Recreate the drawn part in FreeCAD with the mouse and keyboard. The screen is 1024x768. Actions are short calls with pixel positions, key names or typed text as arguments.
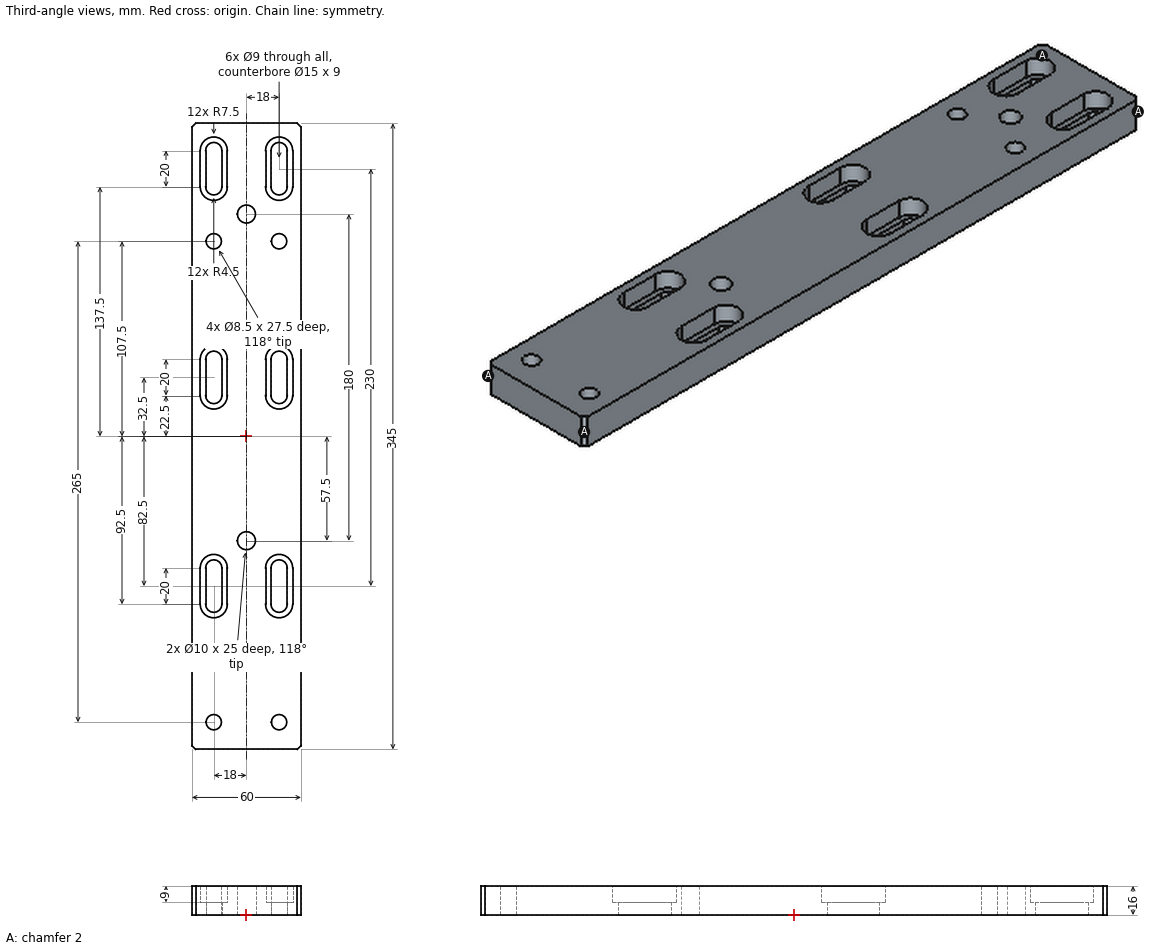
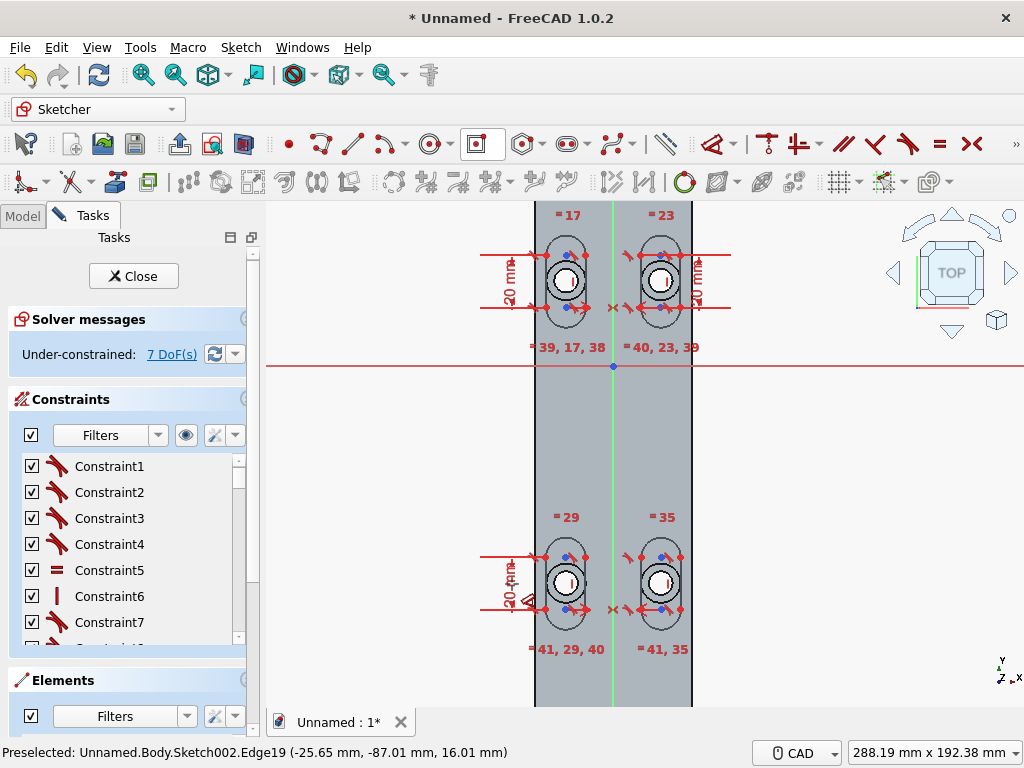
click(641, 594)
click(699, 584)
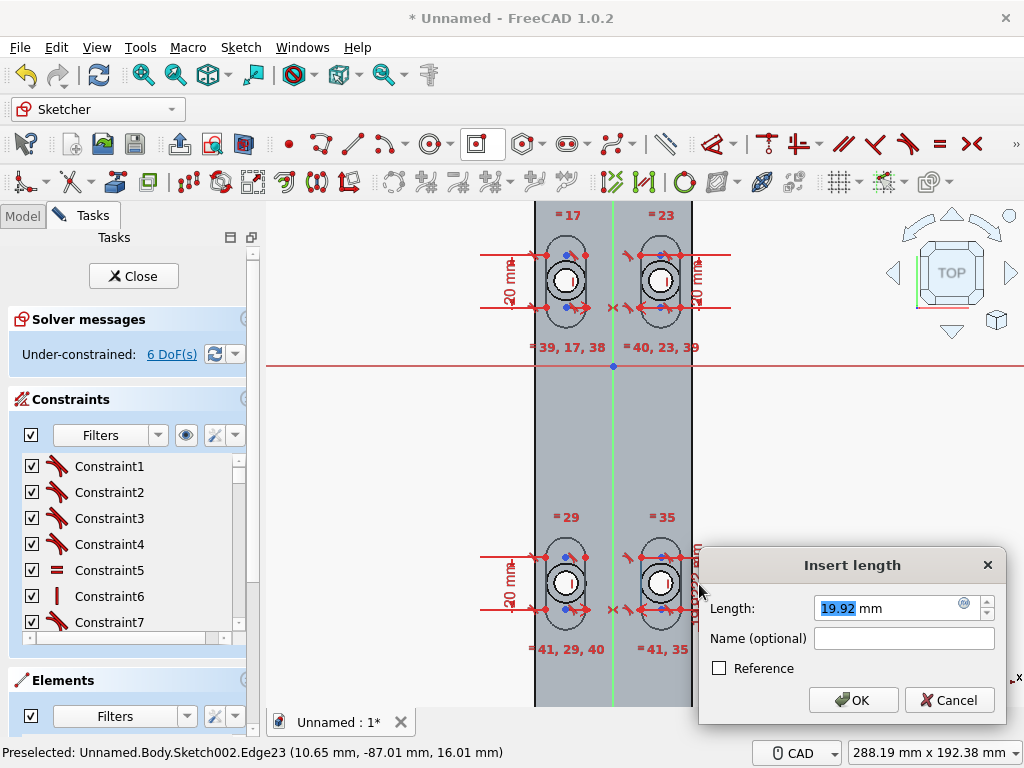
text(20)
key(Return)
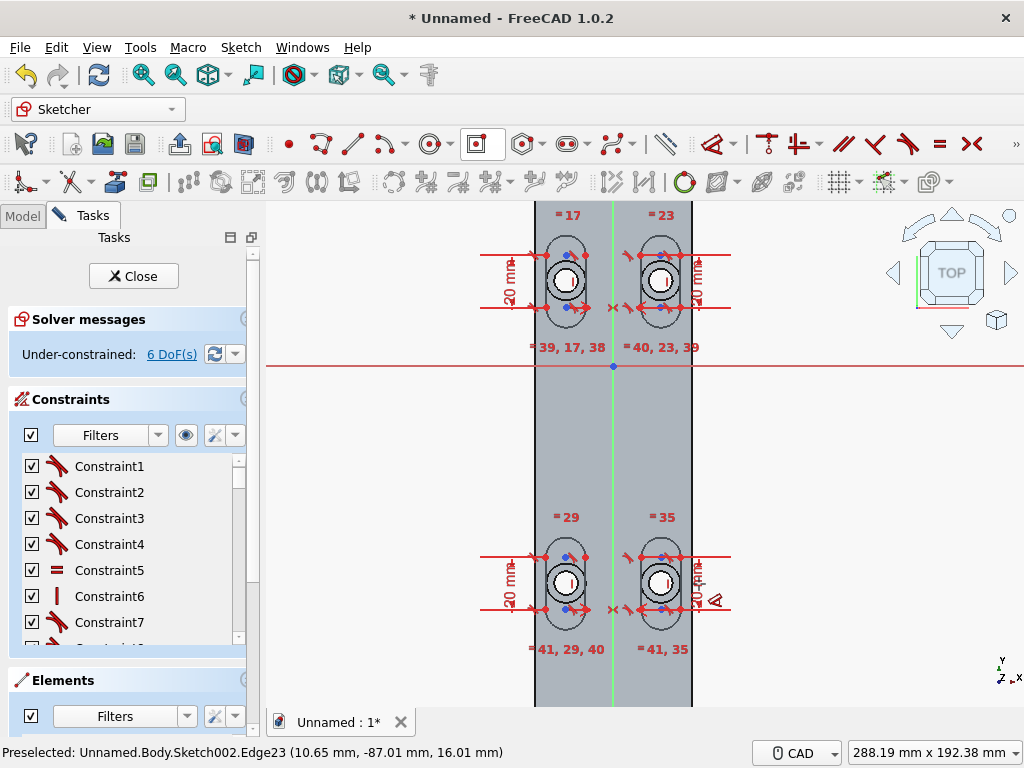
scroll(546, 595, down, 4)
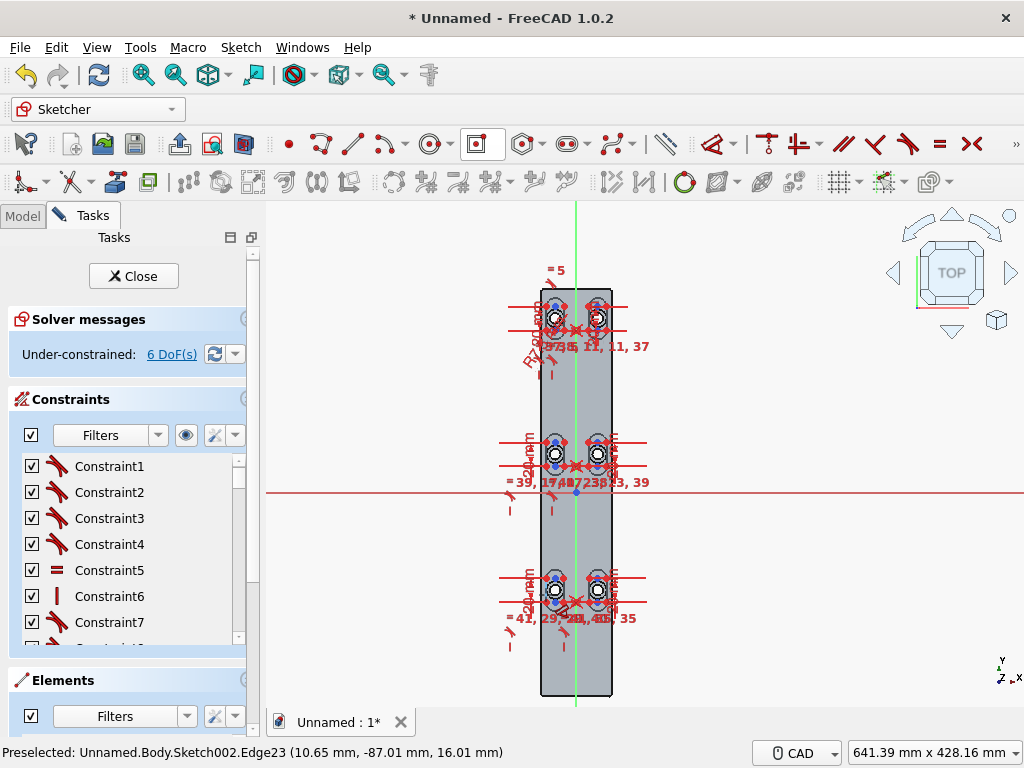
scroll(555, 331, up, 4)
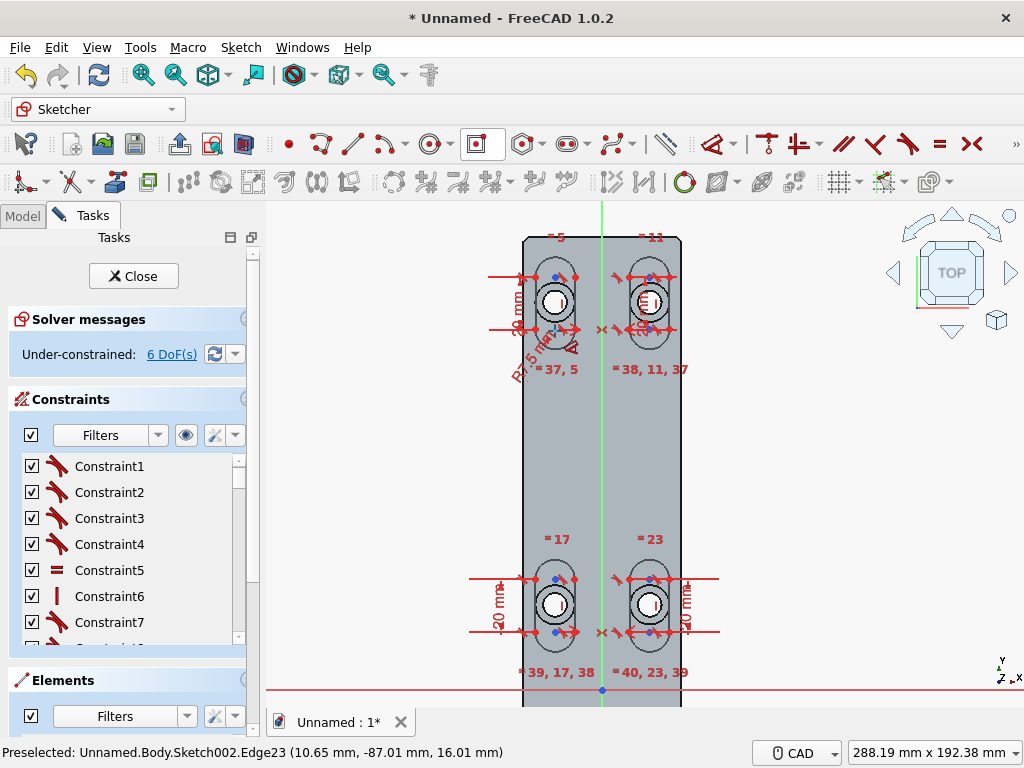
click(555, 330)
click(579, 248)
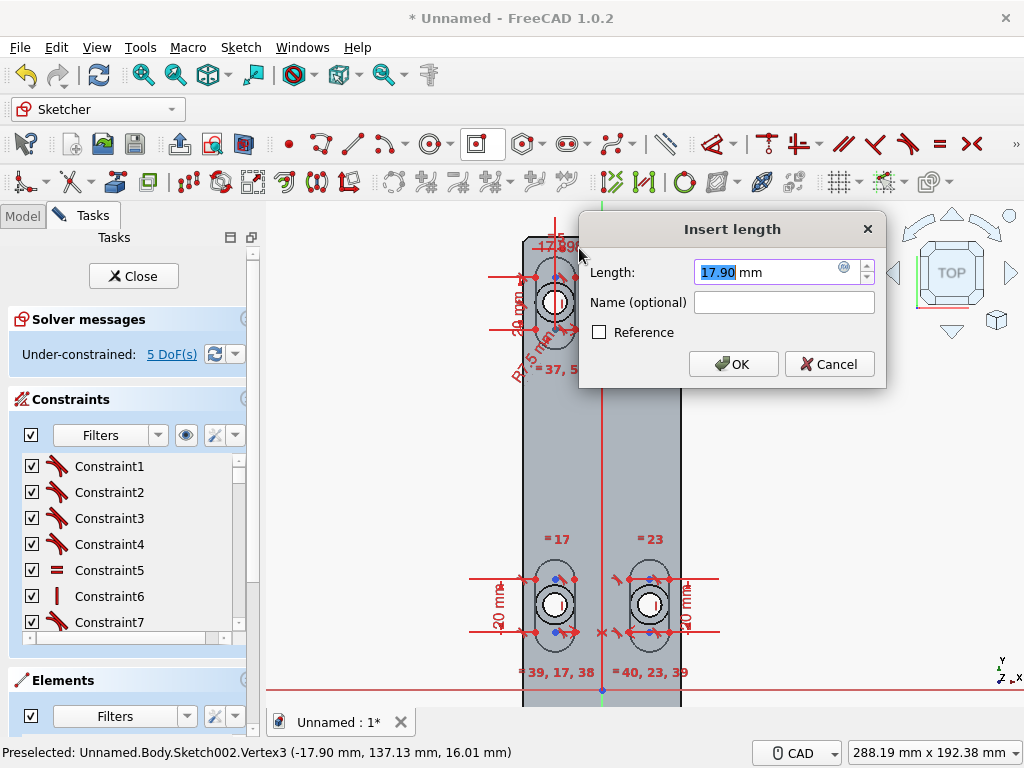
text(18)
key(Return)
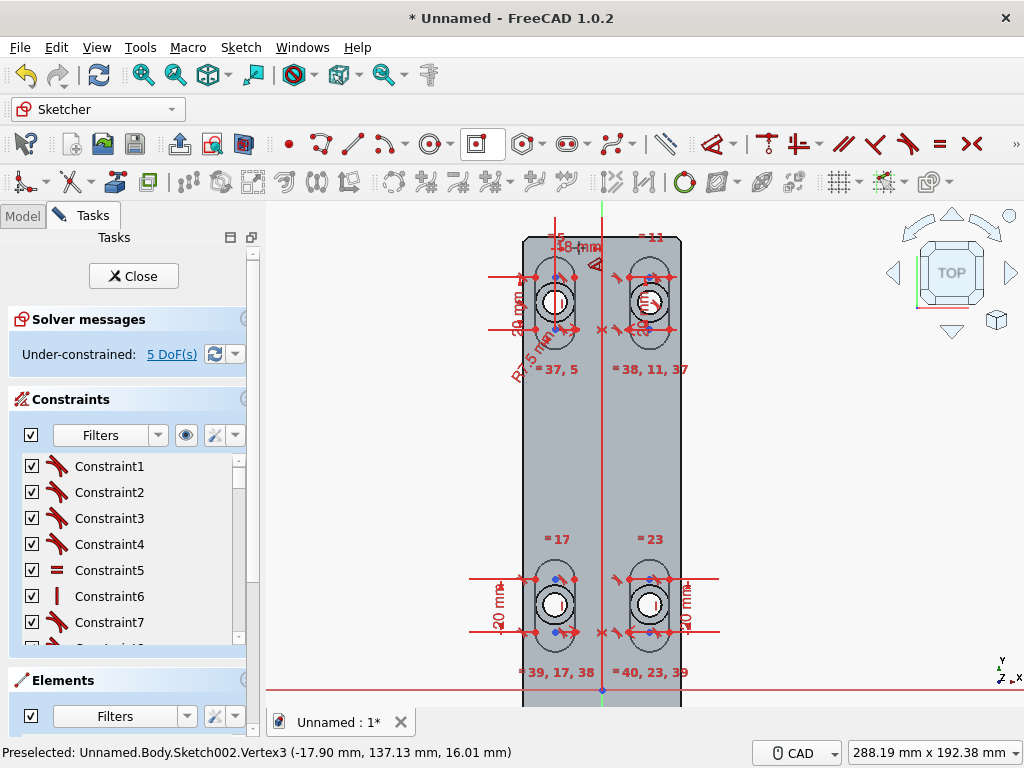
click(555, 632)
click(579, 550)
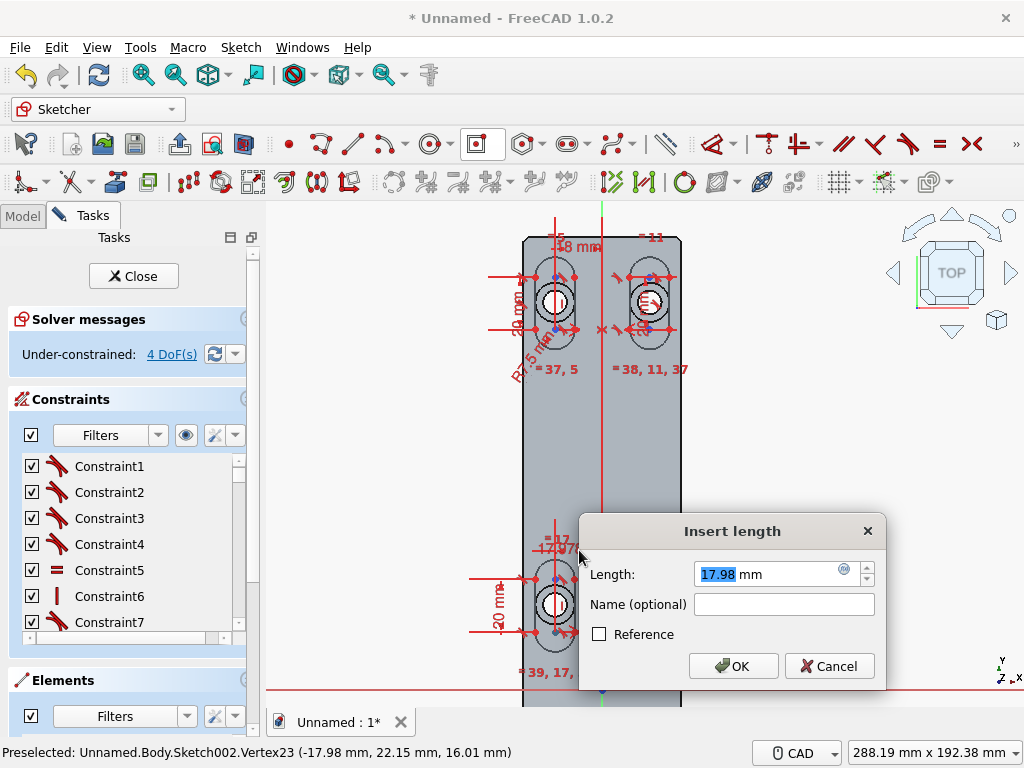
text(18)
key(Return)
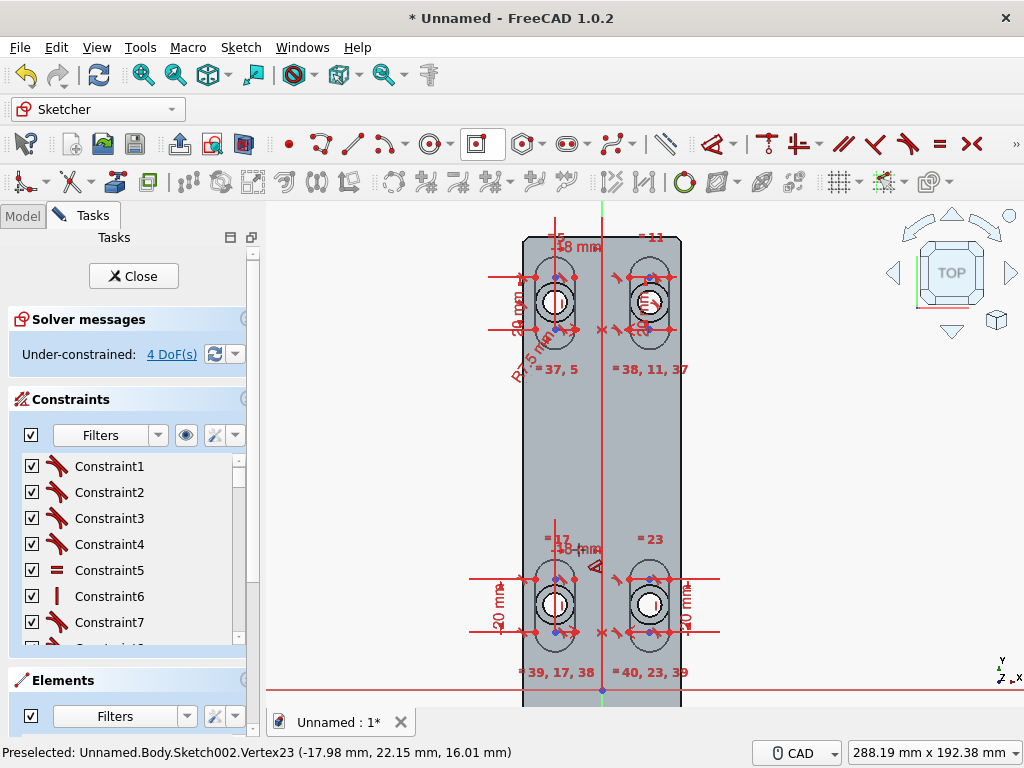
scroll(555, 331, down, 4)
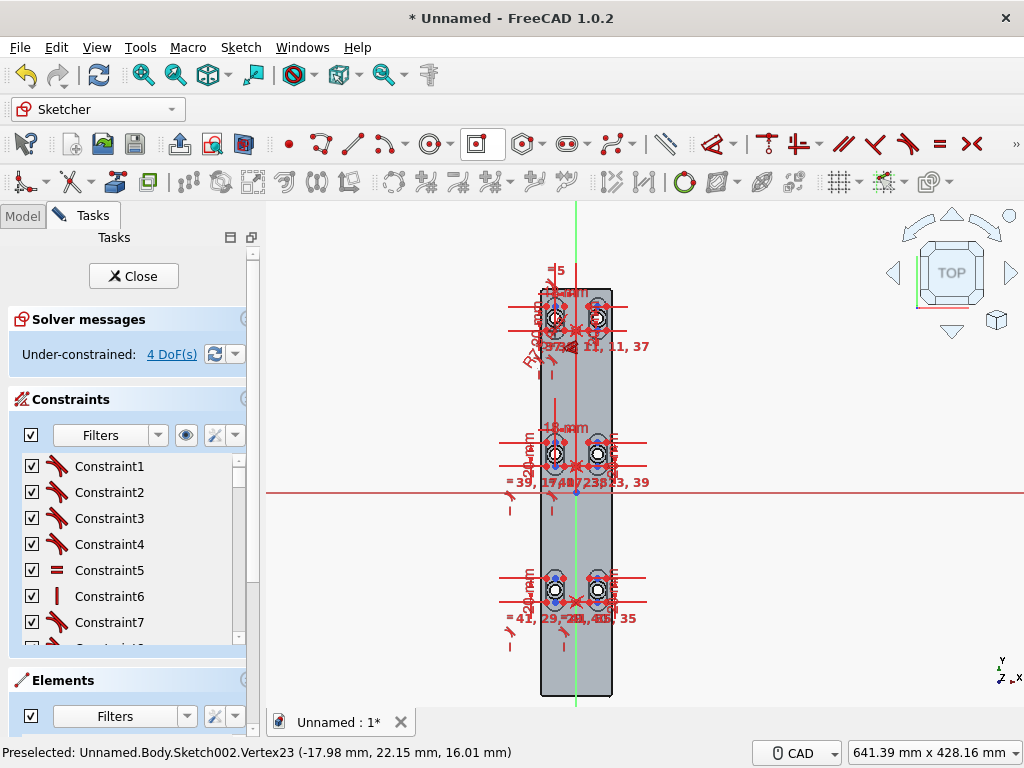
scroll(555, 602, up, 4)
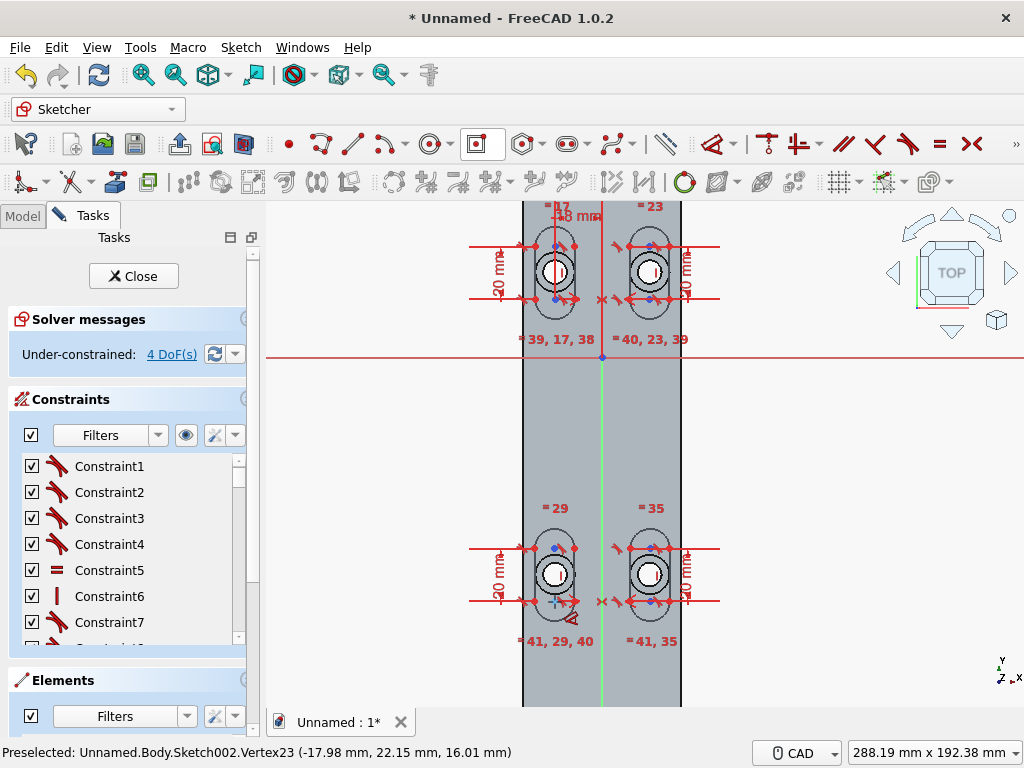
click(555, 601)
click(579, 635)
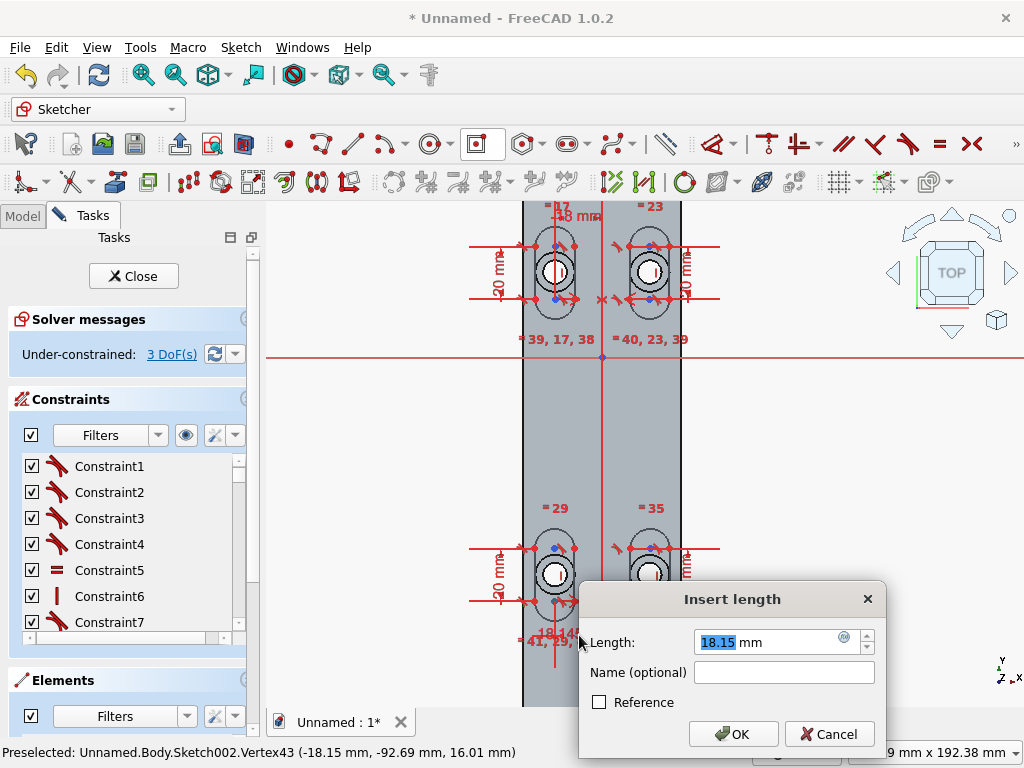
text(18)
key(Return)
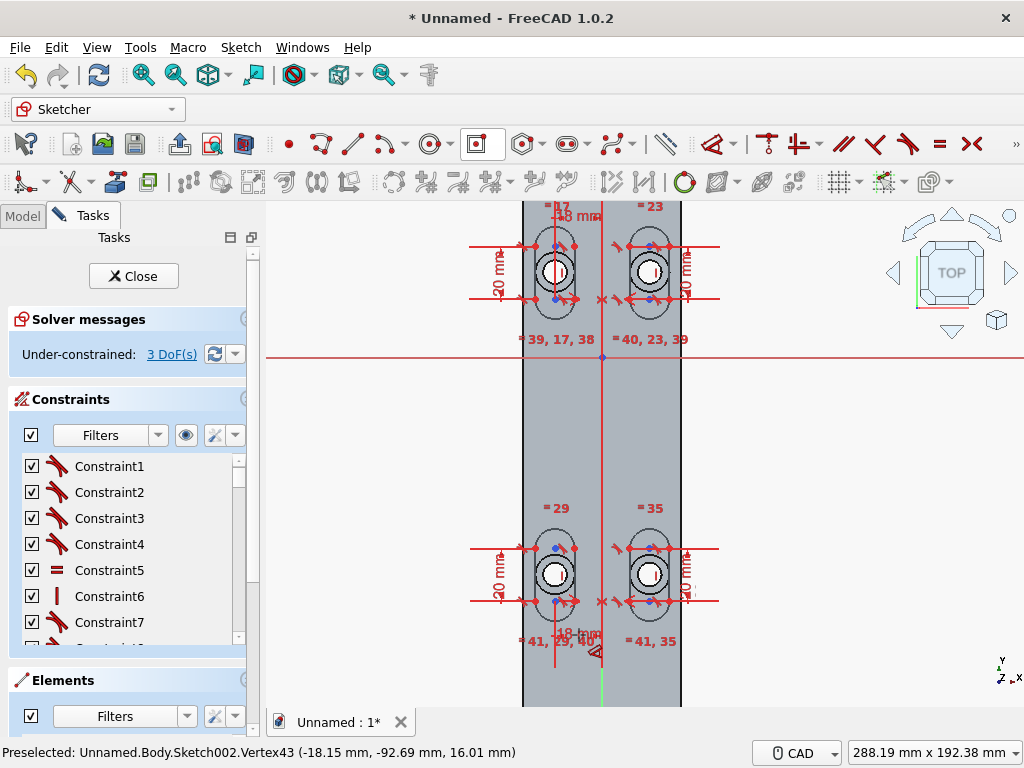
click(535, 299)
click(501, 328)